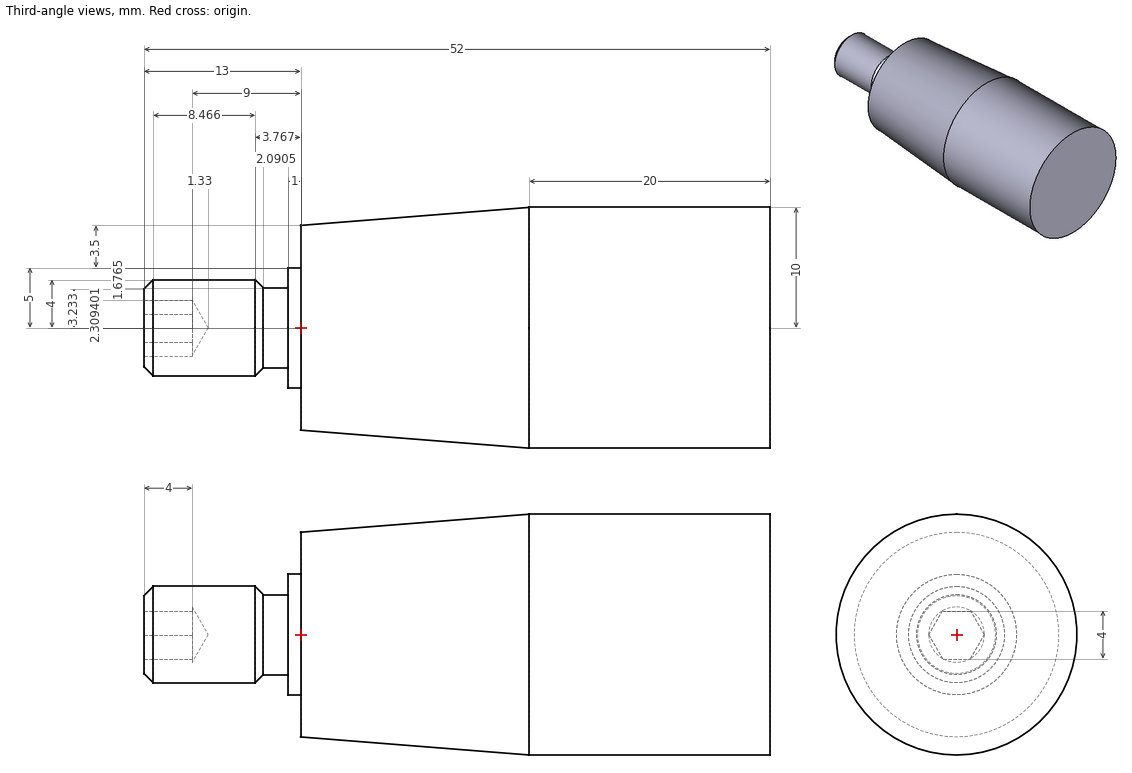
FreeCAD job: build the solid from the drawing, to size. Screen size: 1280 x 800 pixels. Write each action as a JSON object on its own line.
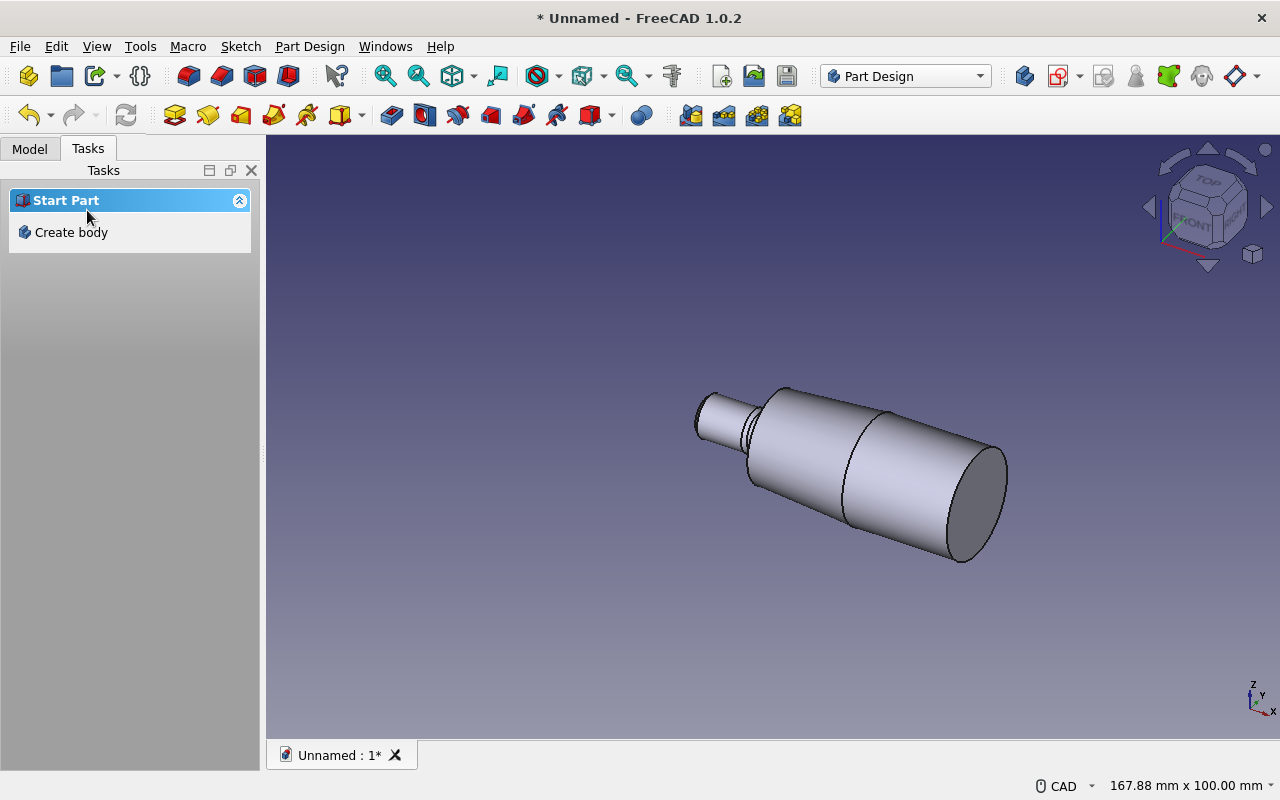
{"action": "left_click", "coordinate": [386, 76]}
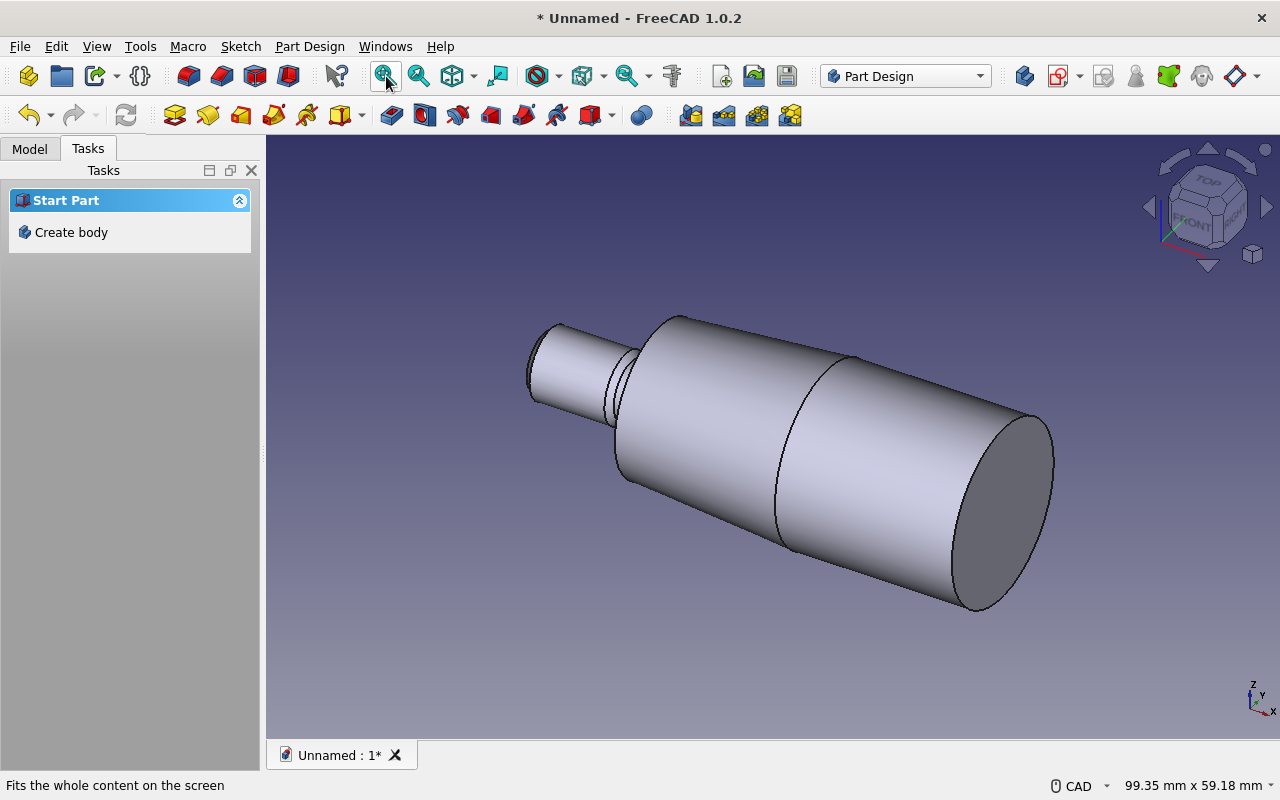
{"action": "key", "text": "6"}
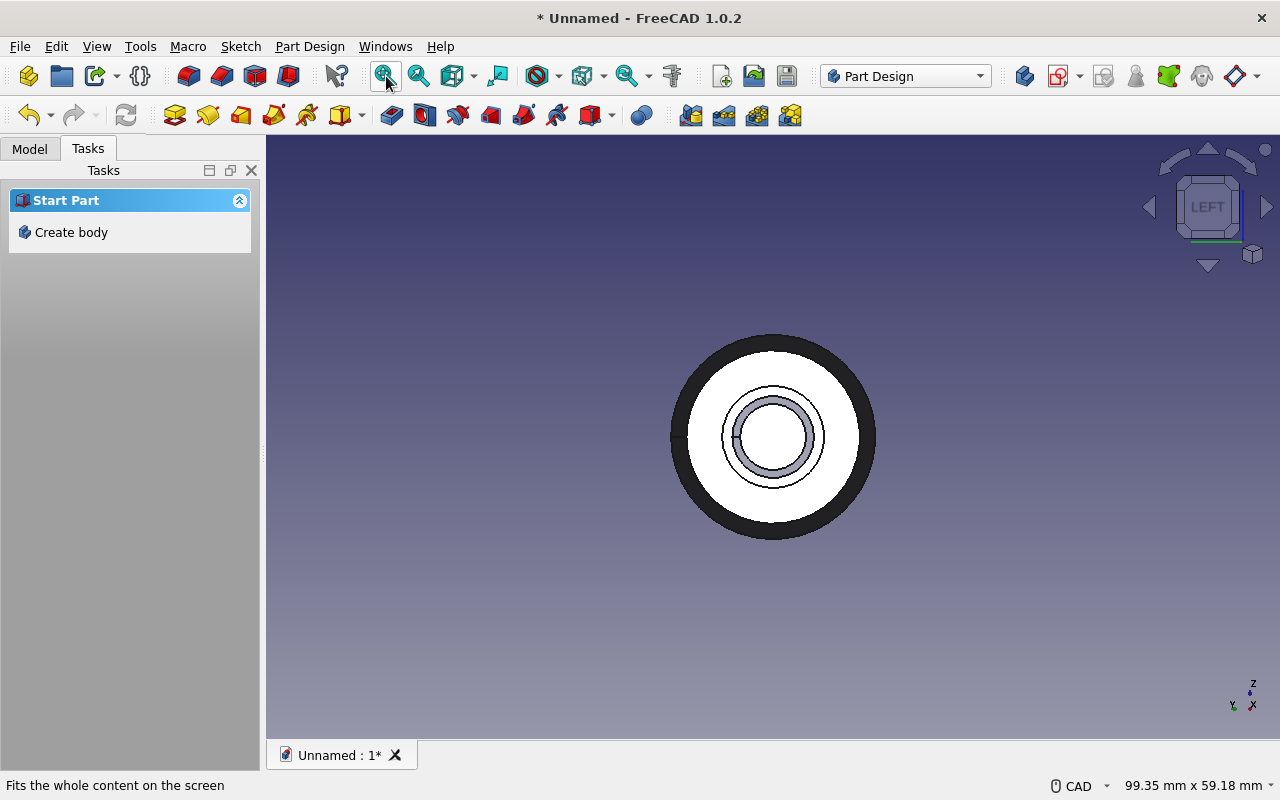
{"action": "left_click", "coordinate": [386, 76]}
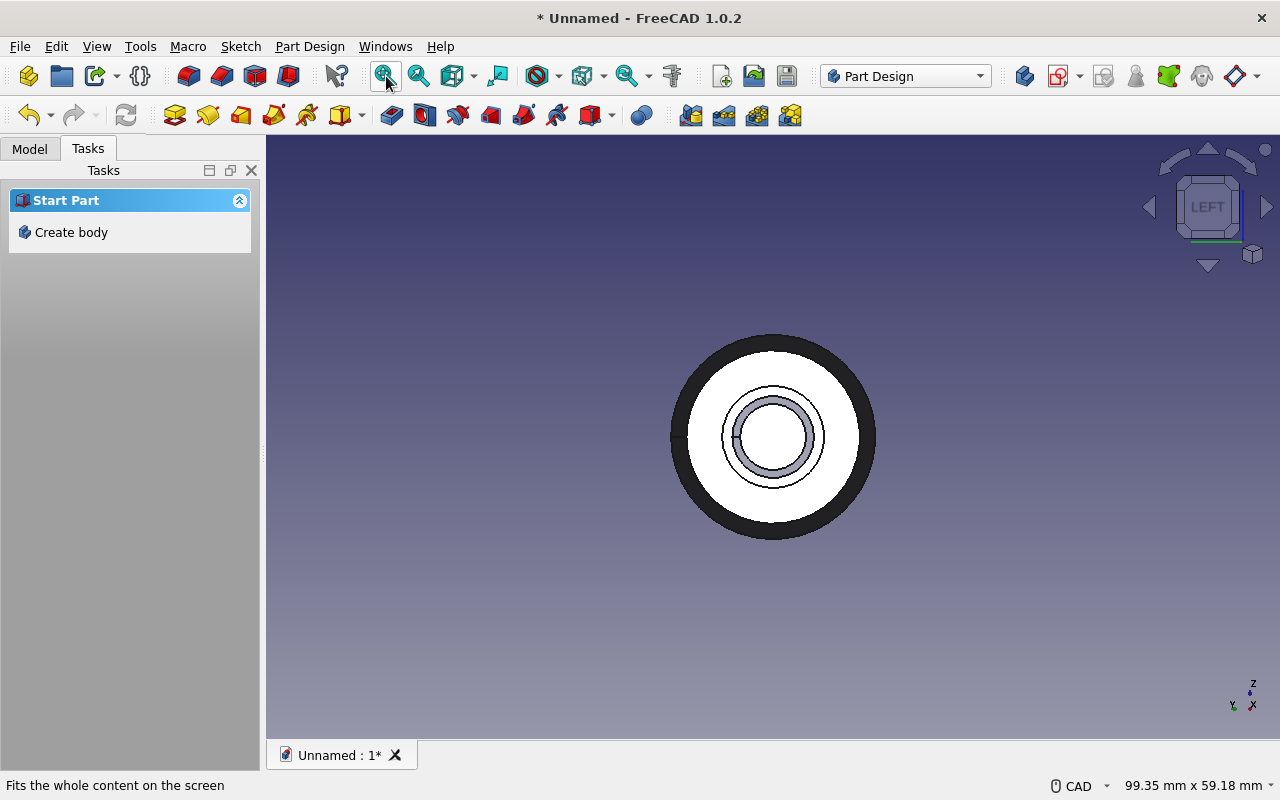
{"action": "left_click", "coordinate": [773, 436]}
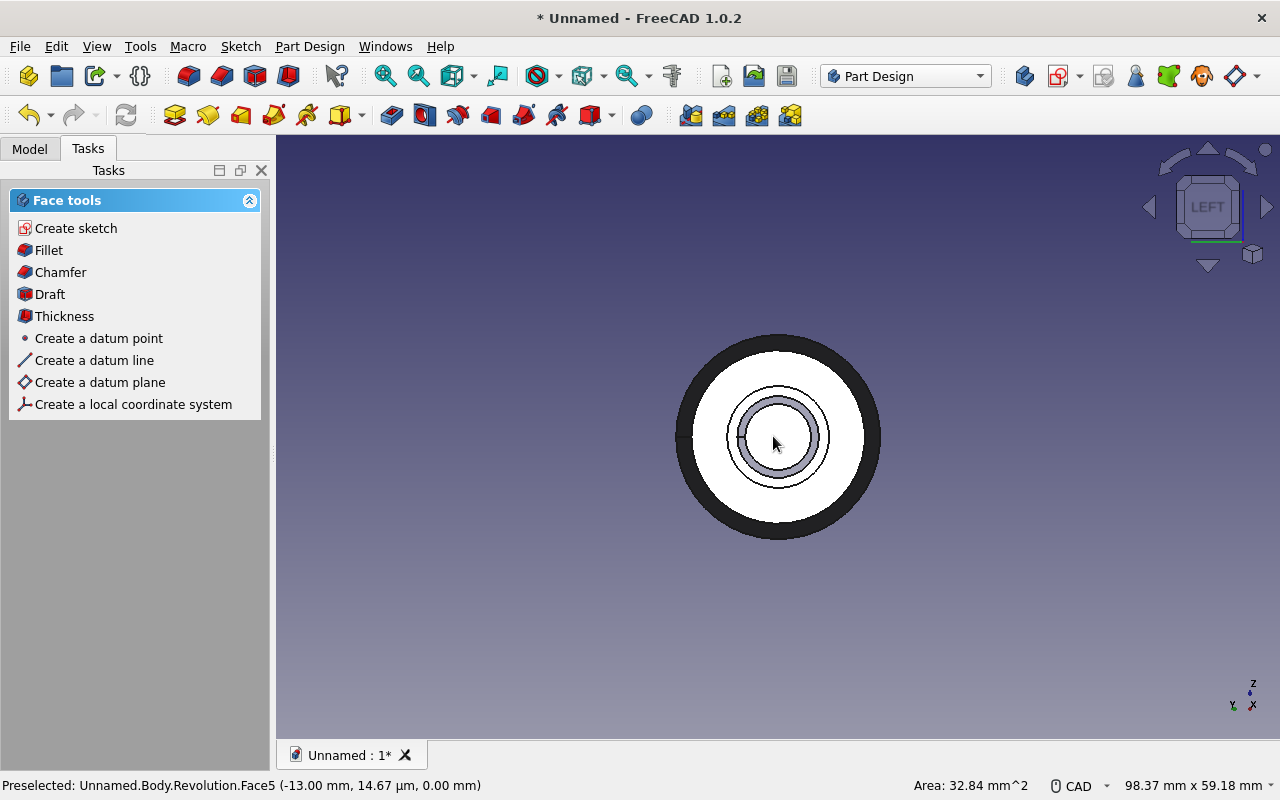
{"action": "left_click", "coordinate": [1058, 76]}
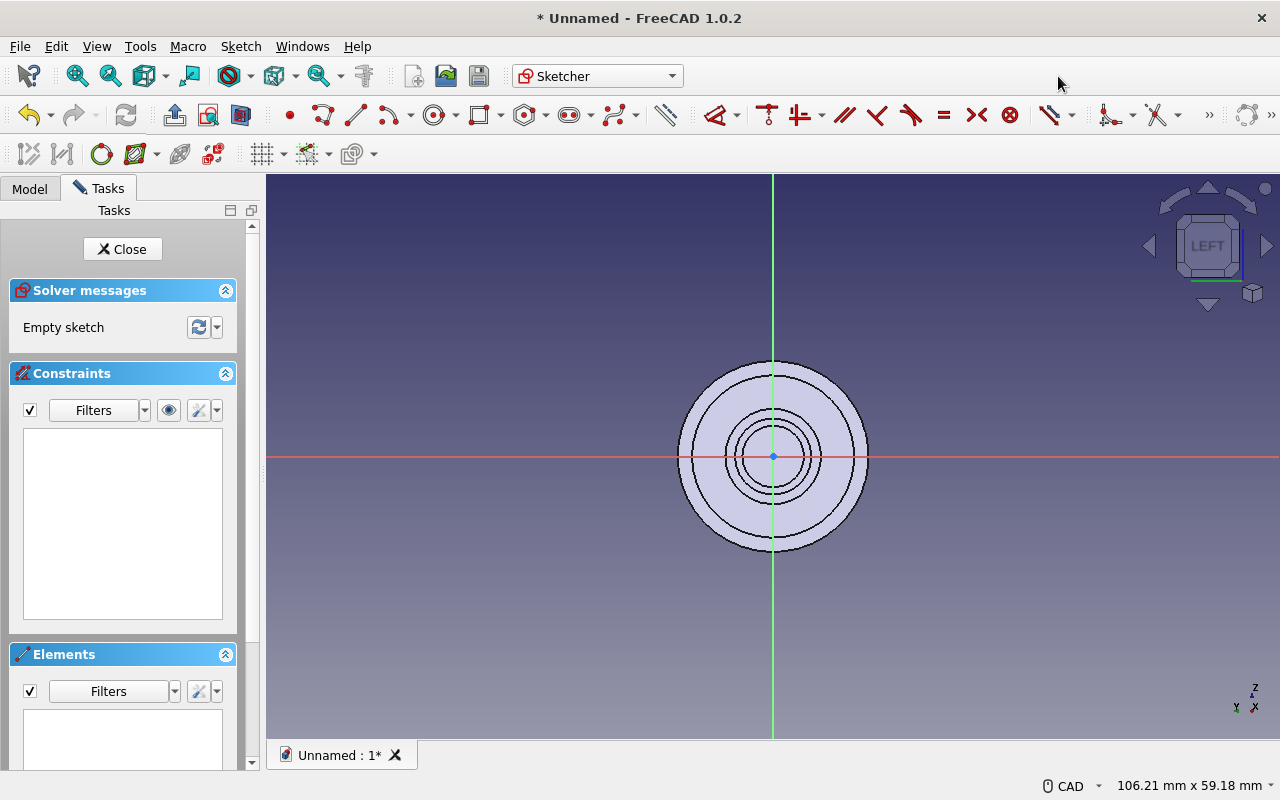
{"action": "scroll", "coordinate": [782, 456], "scroll_direction": "up", "scroll_amount": 11}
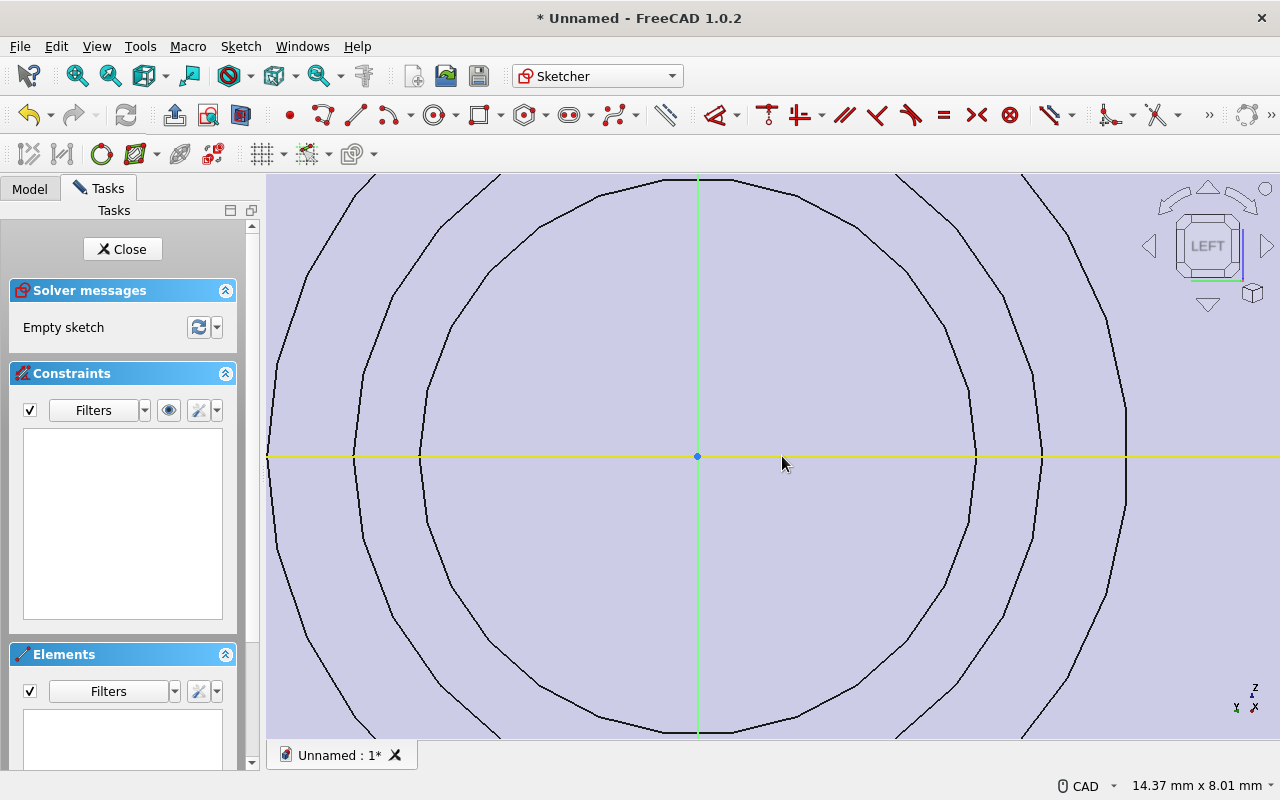
{"action": "key", "text": "g p 6"}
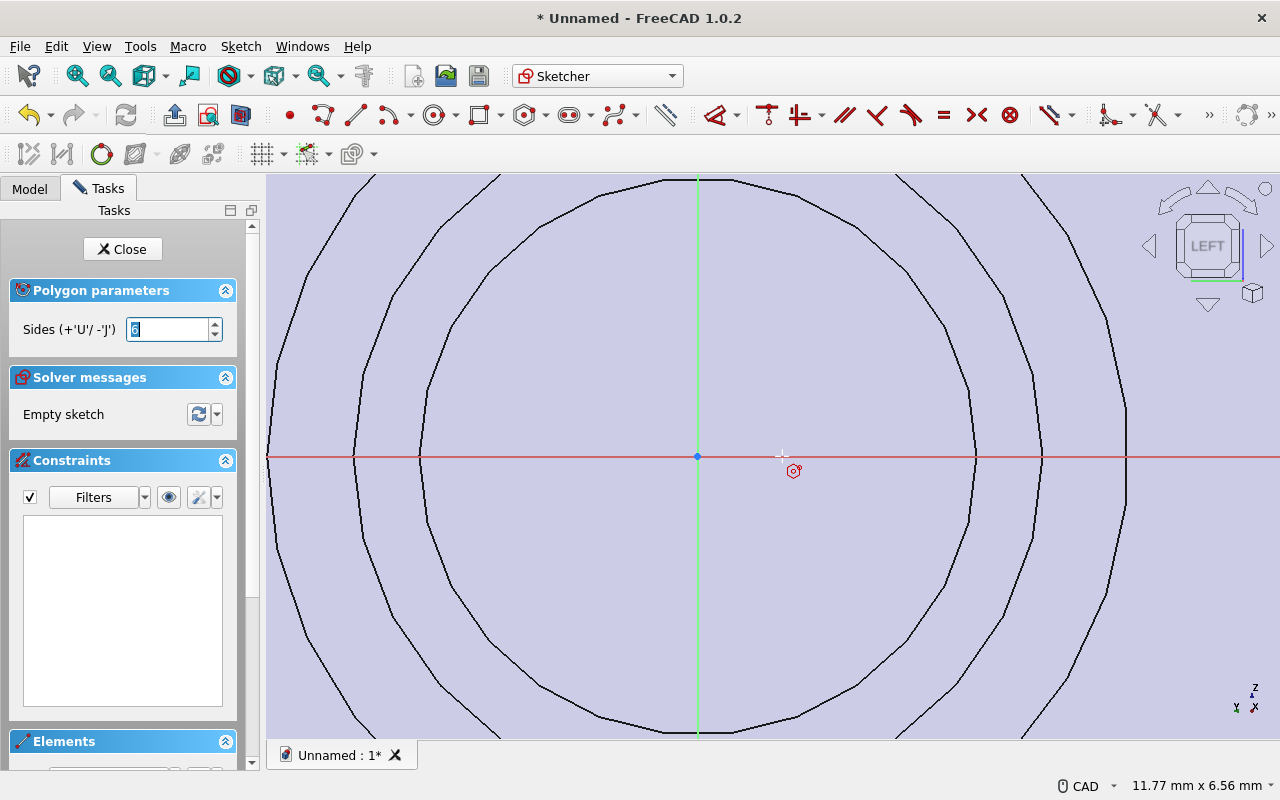
{"action": "left_click", "coordinate": [698, 456]}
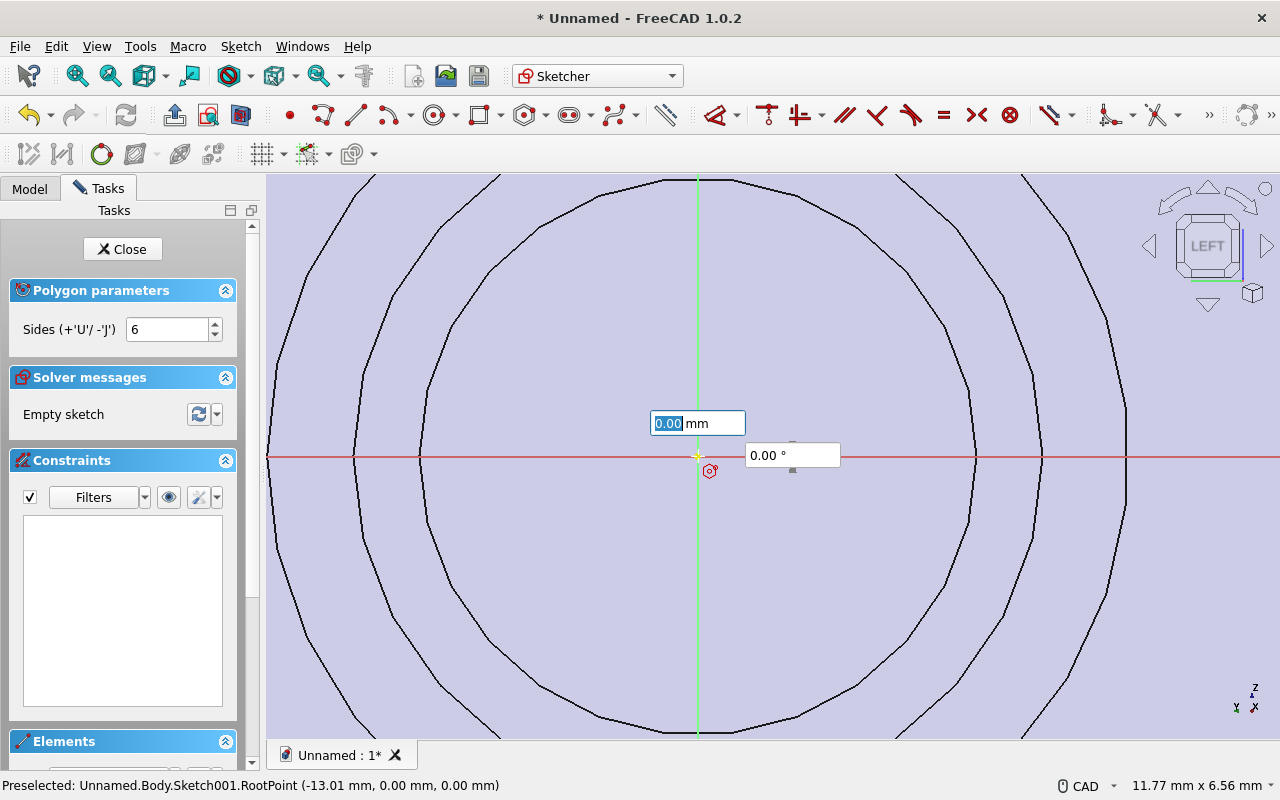
{"action": "left_click", "coordinate": [897, 456]}
{"action": "right_click", "coordinate": [897, 456]}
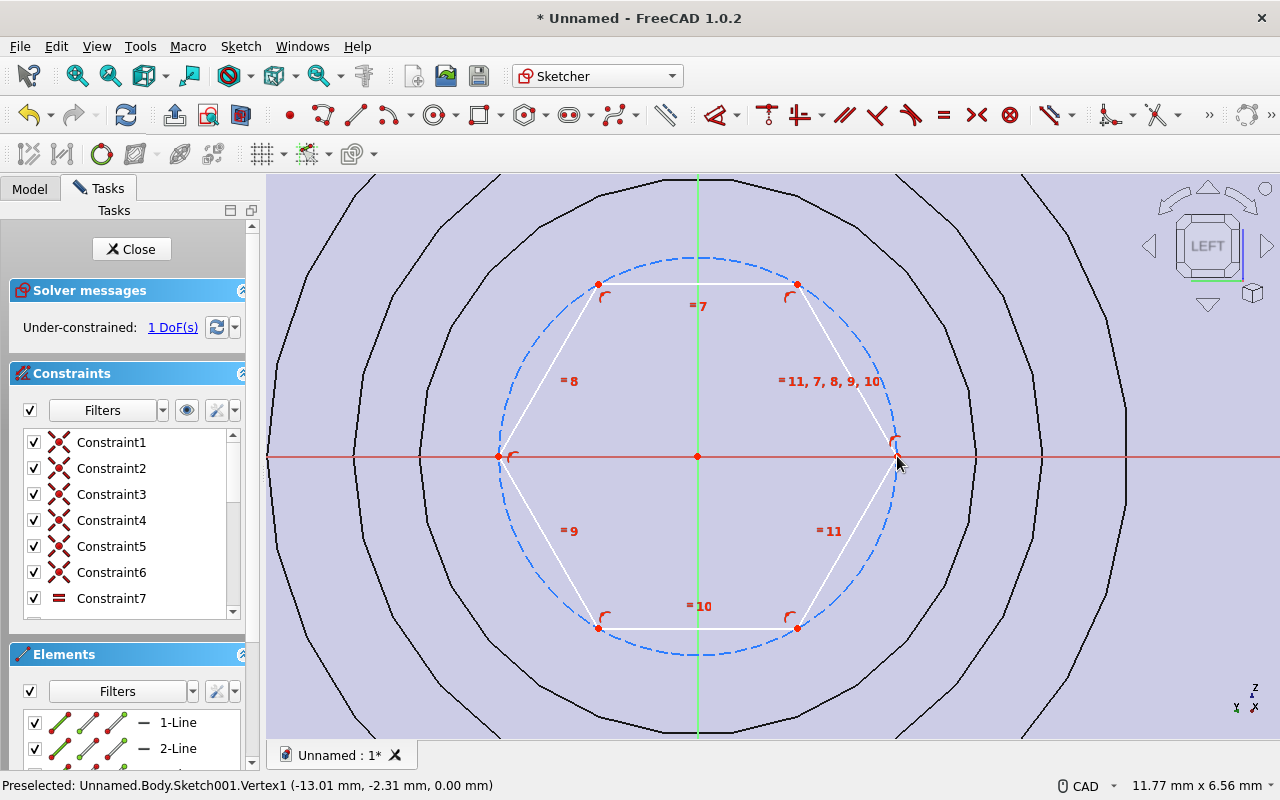
{"action": "left_click", "coordinate": [714, 116]}